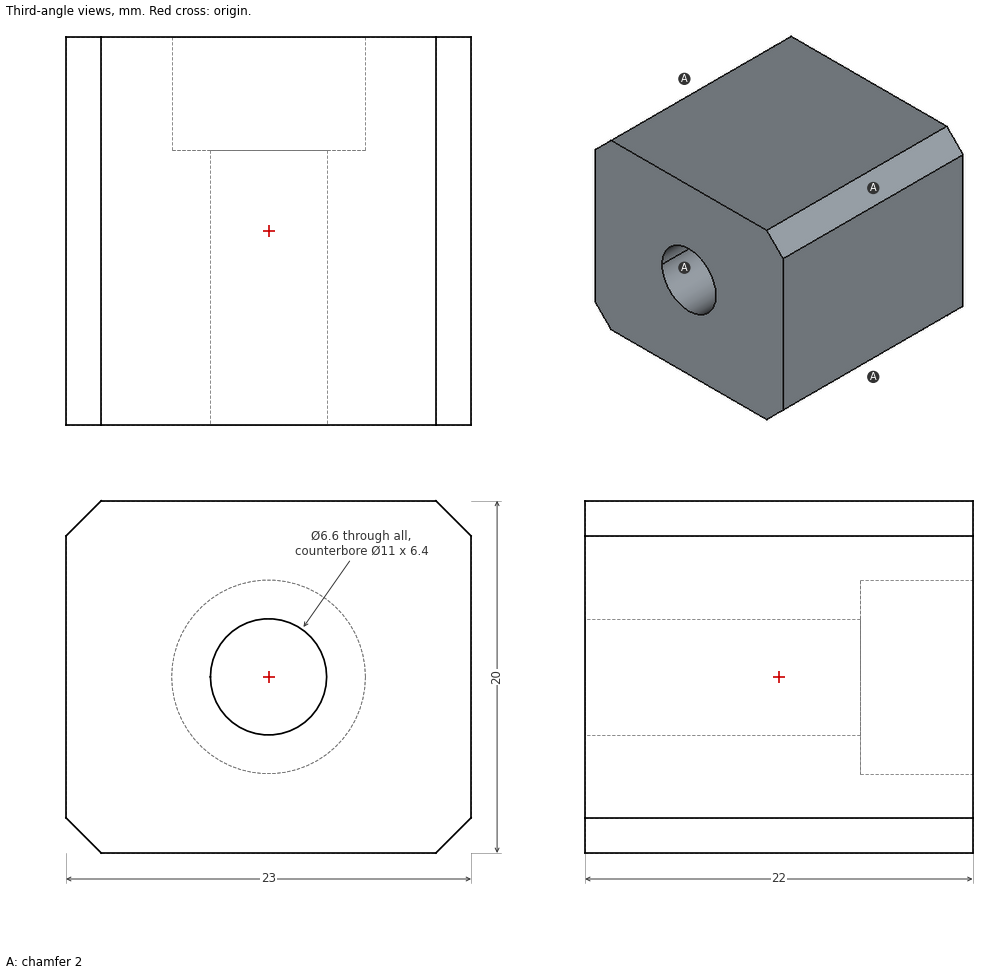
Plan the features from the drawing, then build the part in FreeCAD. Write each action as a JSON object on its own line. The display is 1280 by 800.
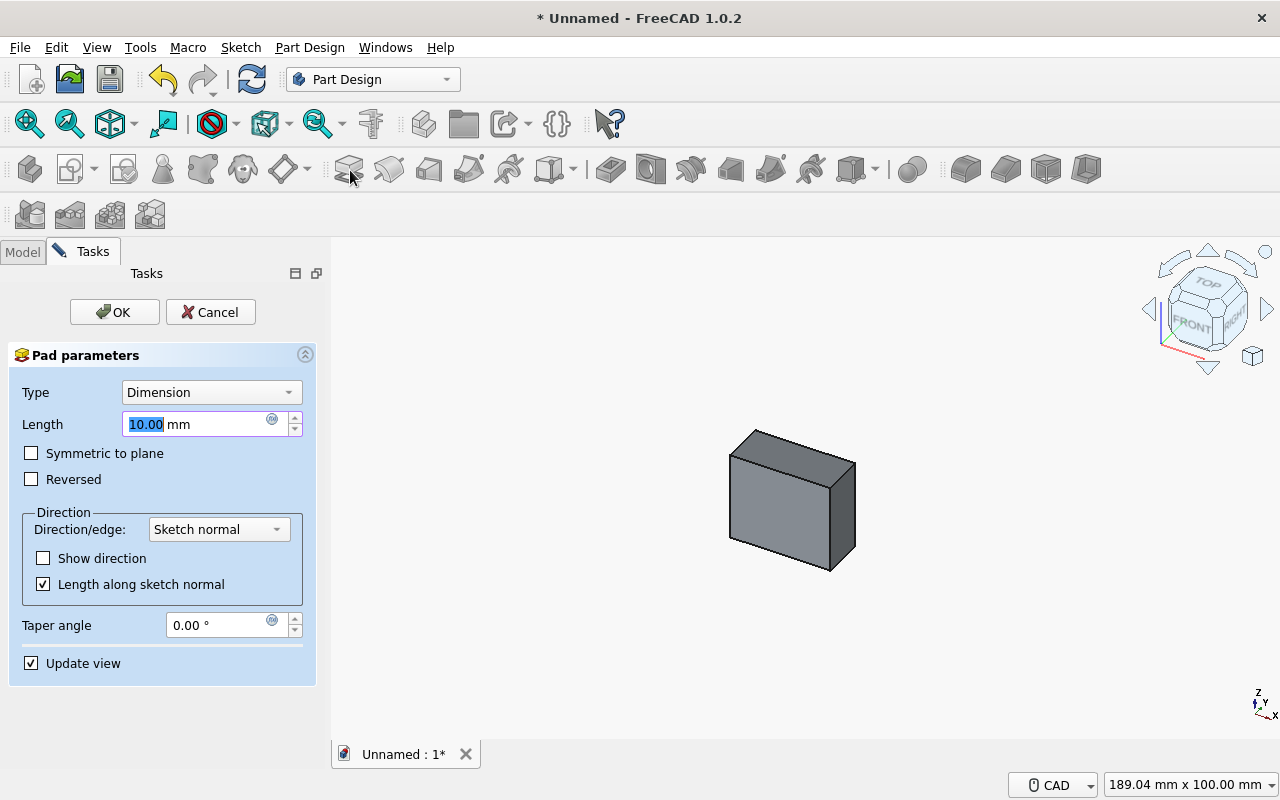
{"action": "type", "text": "22"}
{"action": "key", "text": "Tab"}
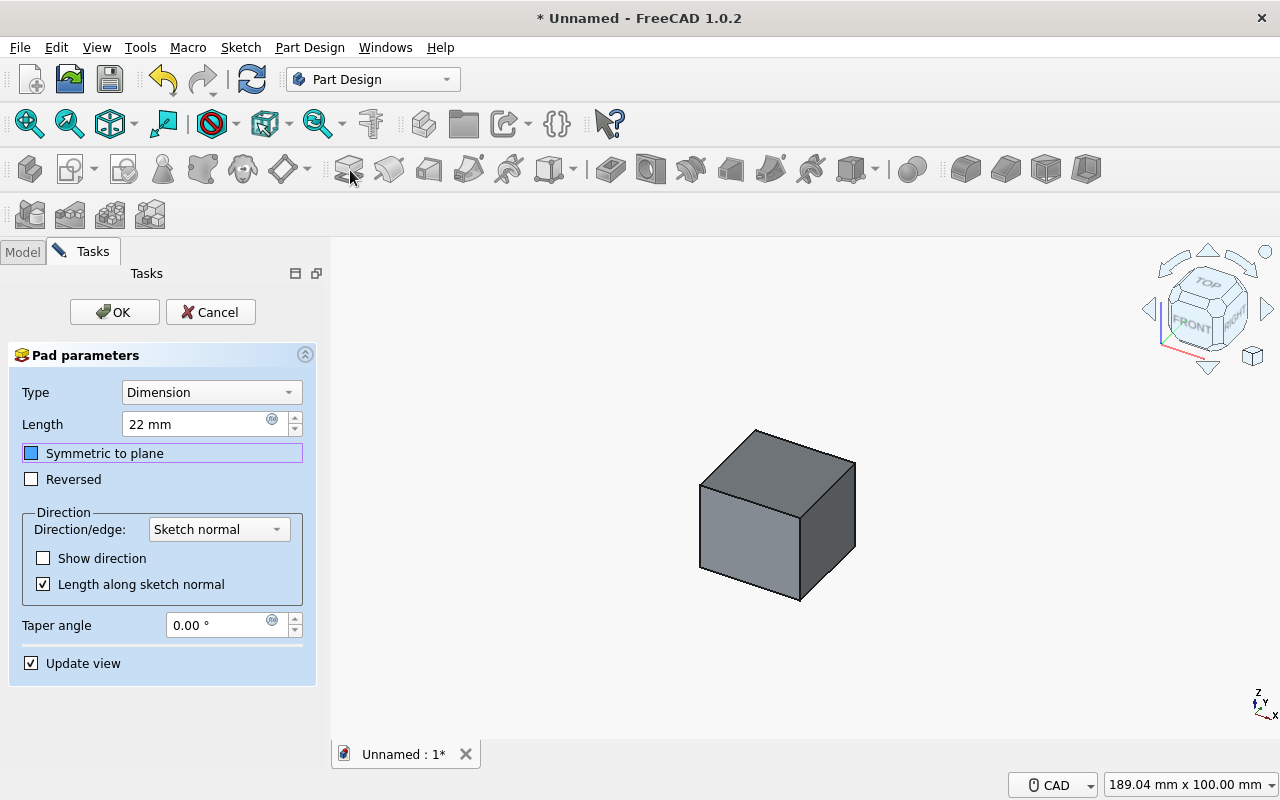
{"action": "left_click", "coordinate": [30, 453]}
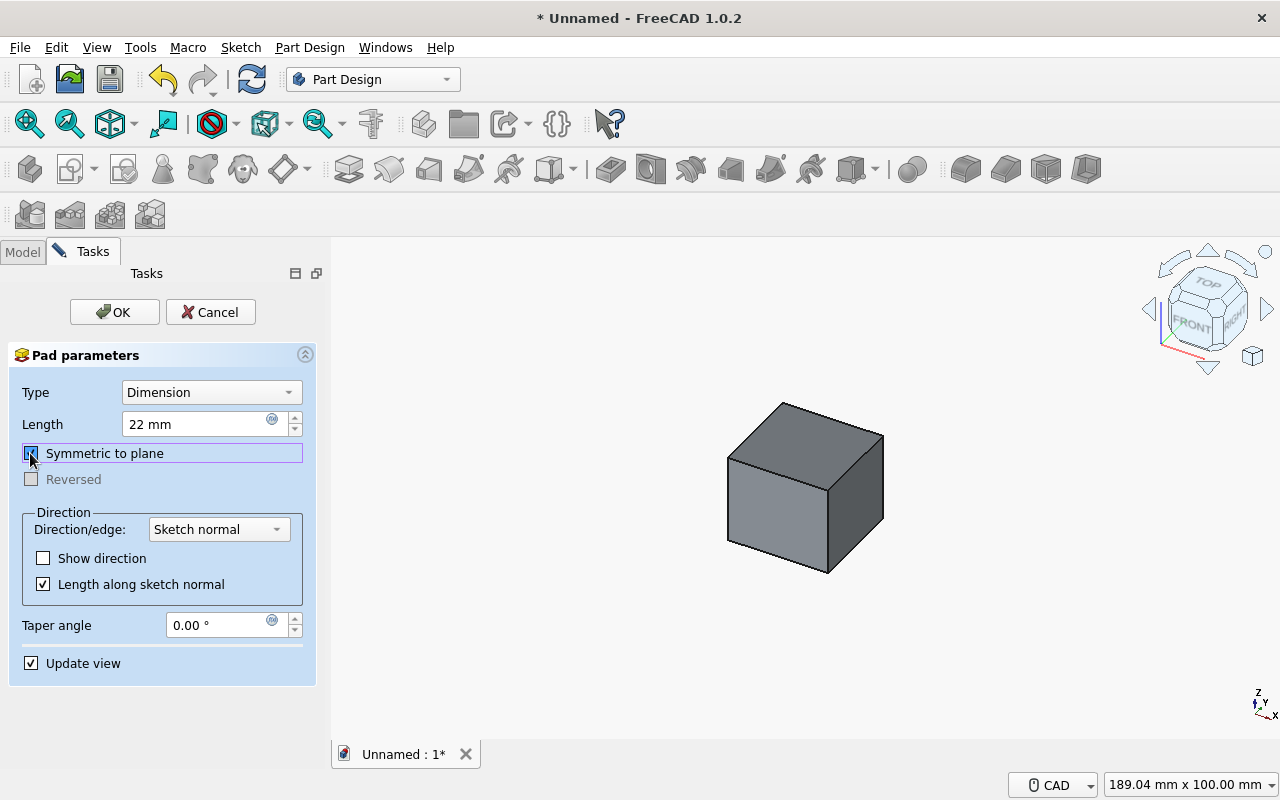
{"action": "left_click", "coordinate": [115, 312]}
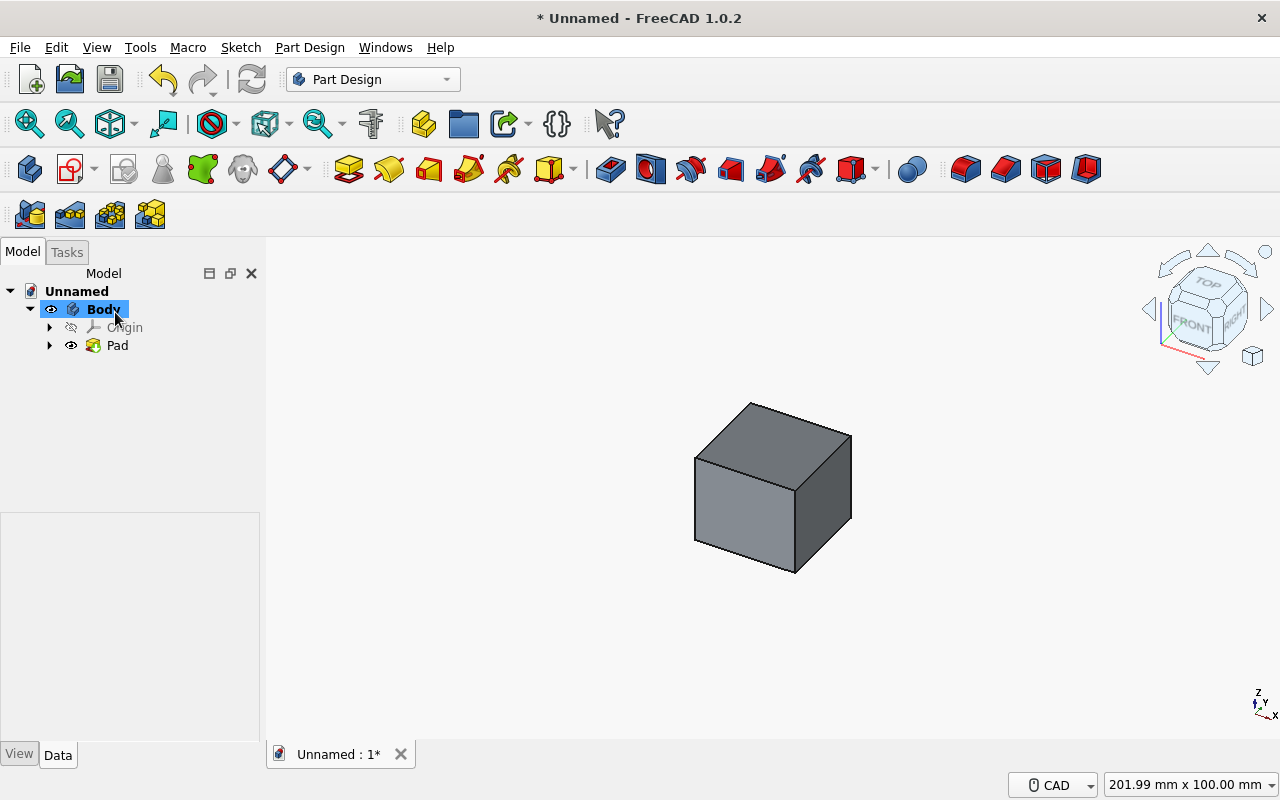
{"action": "key", "text": "v f"}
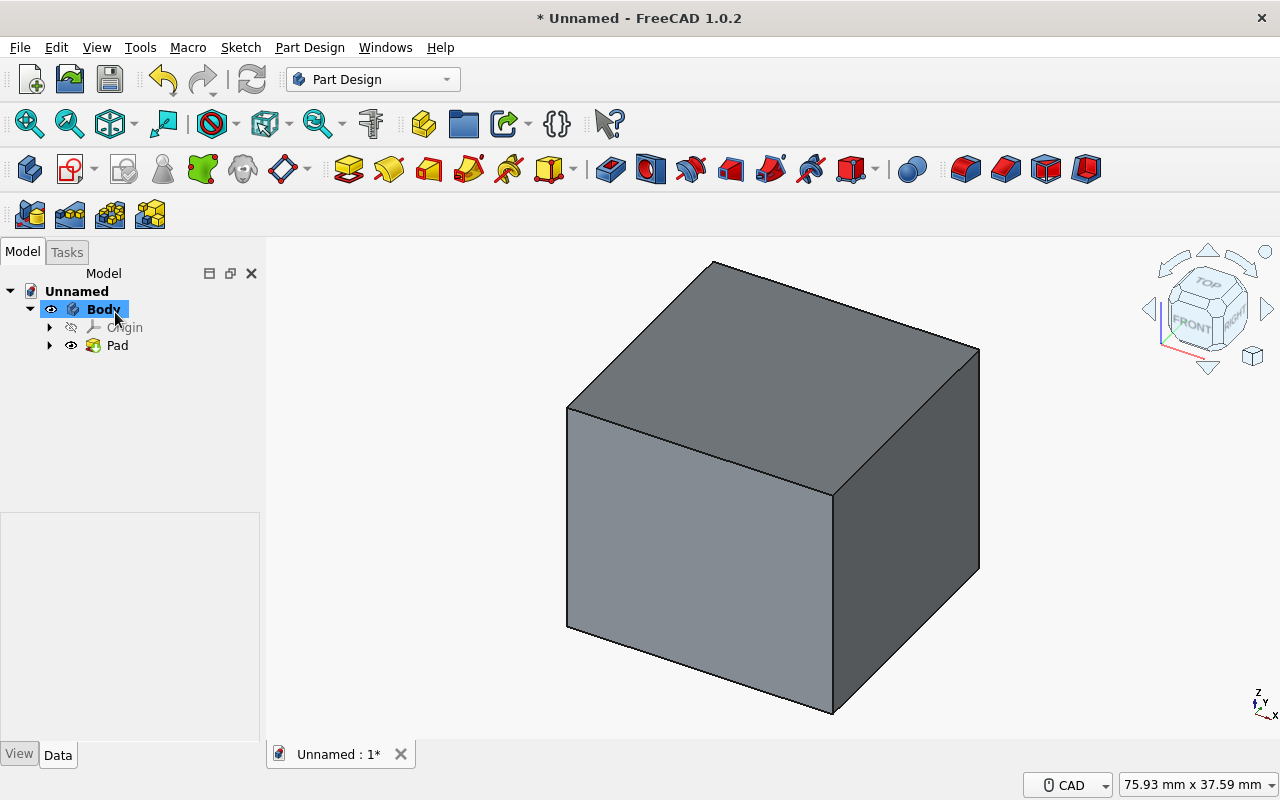
{"action": "key", "text": "4"}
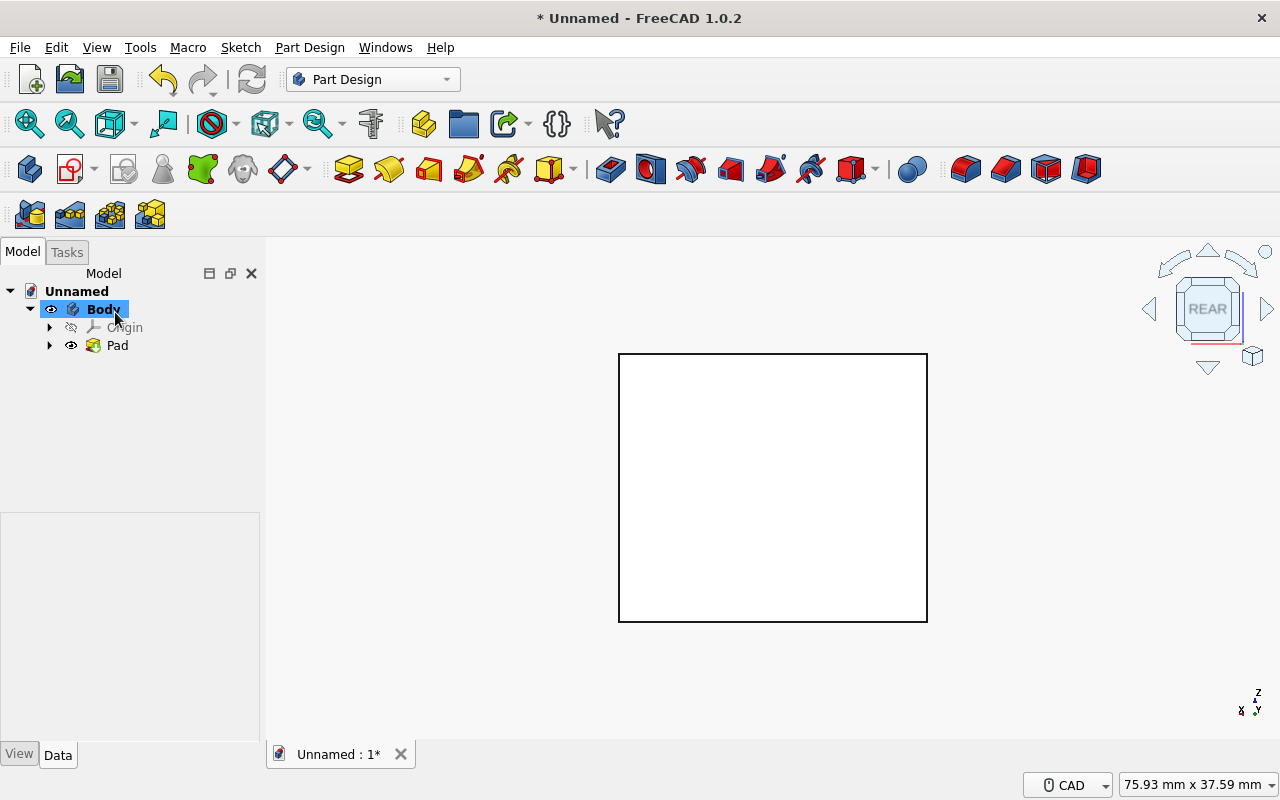
{"action": "left_click", "coordinate": [773, 487]}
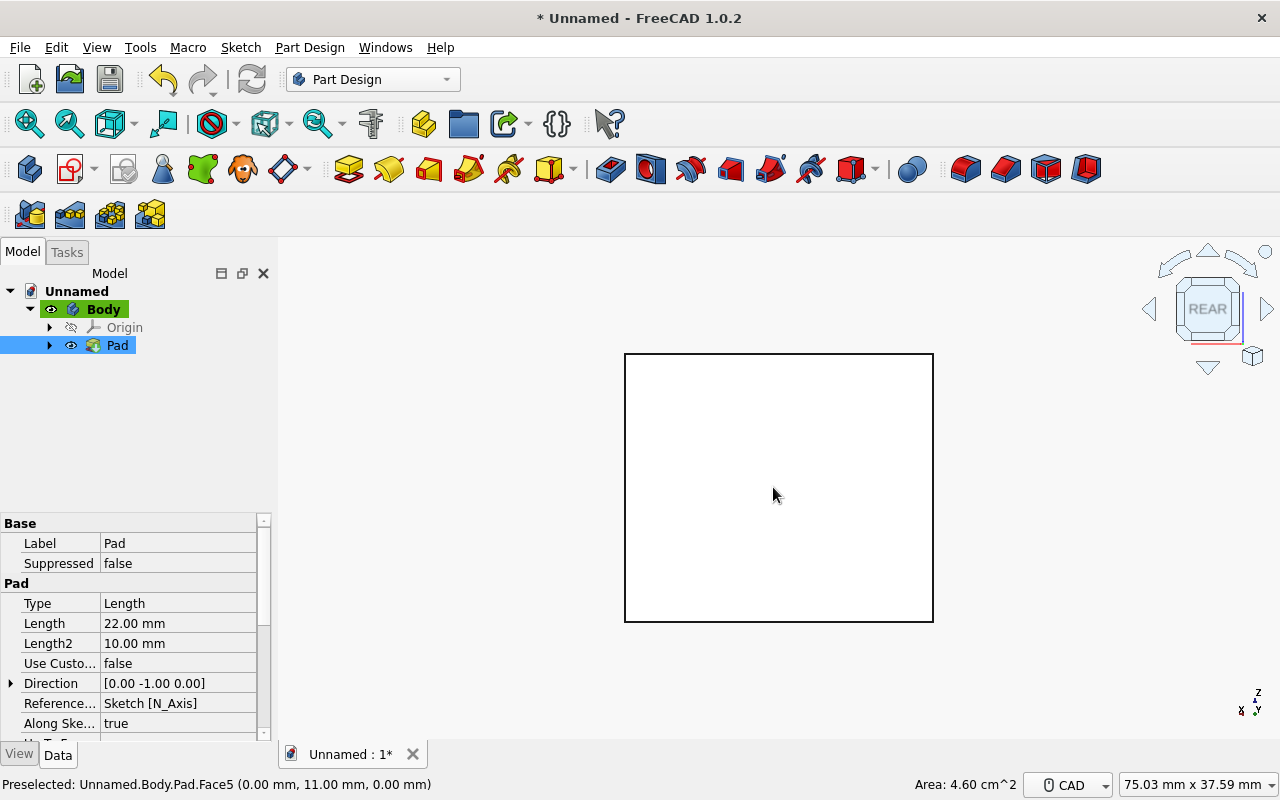
{"action": "left_click", "coordinate": [70, 170]}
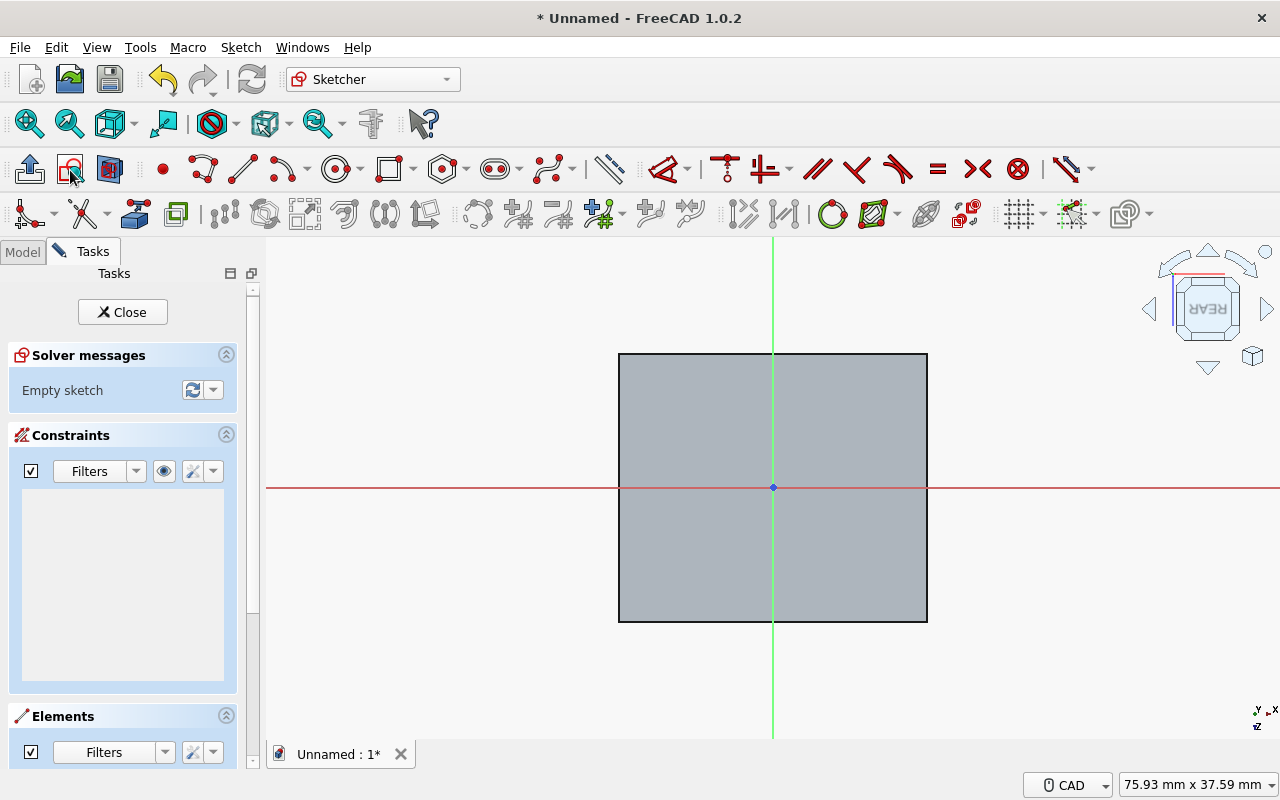
{"action": "scroll", "coordinate": [803, 488], "scroll_direction": "up", "scroll_amount": 6}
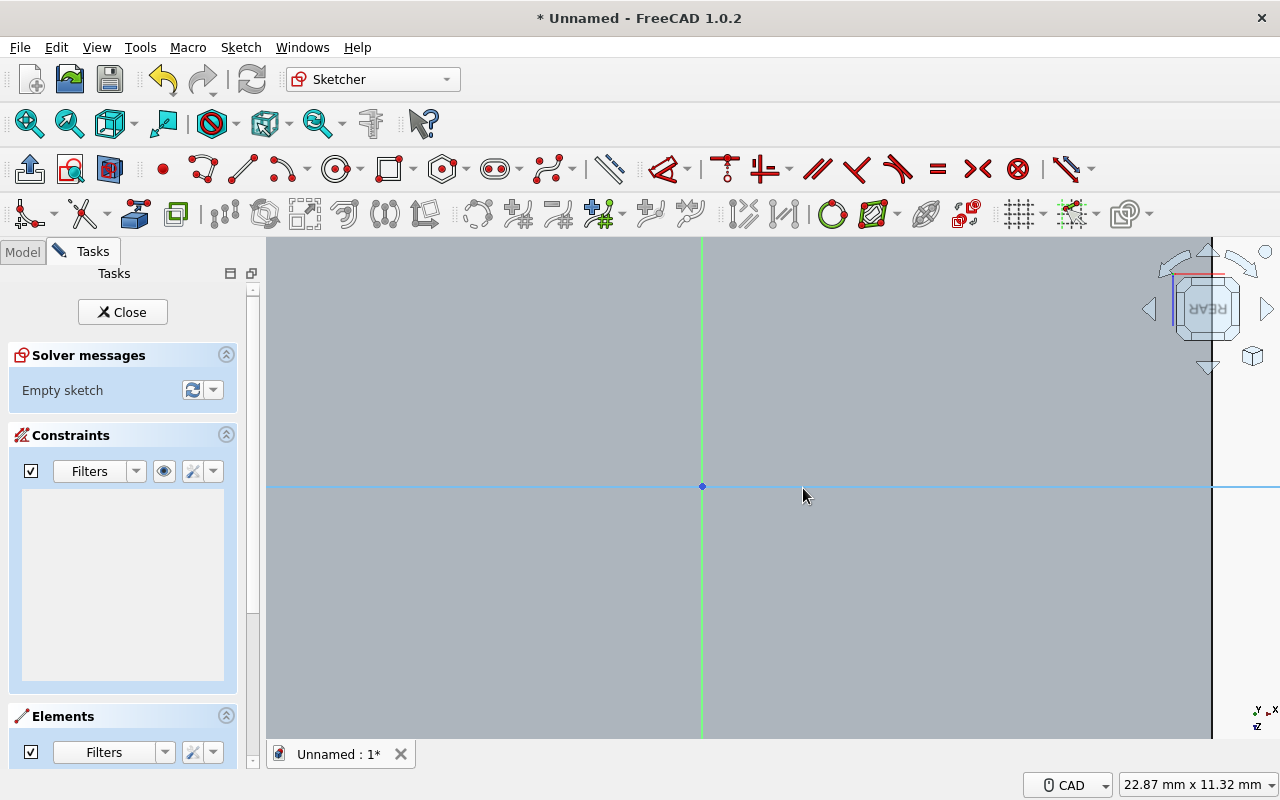
{"action": "key", "text": "g c"}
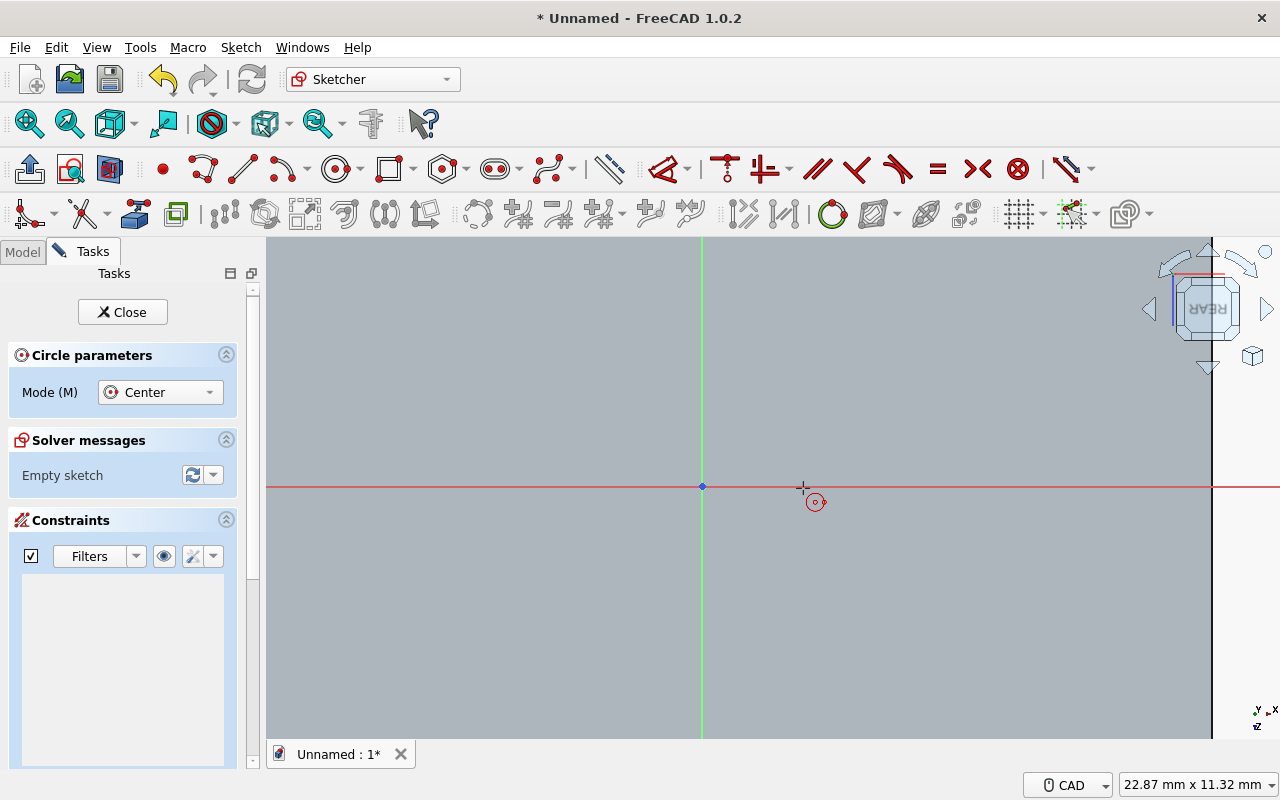
{"action": "left_click", "coordinate": [702, 487]}
{"action": "mouse_move", "coordinate": [806, 383]}